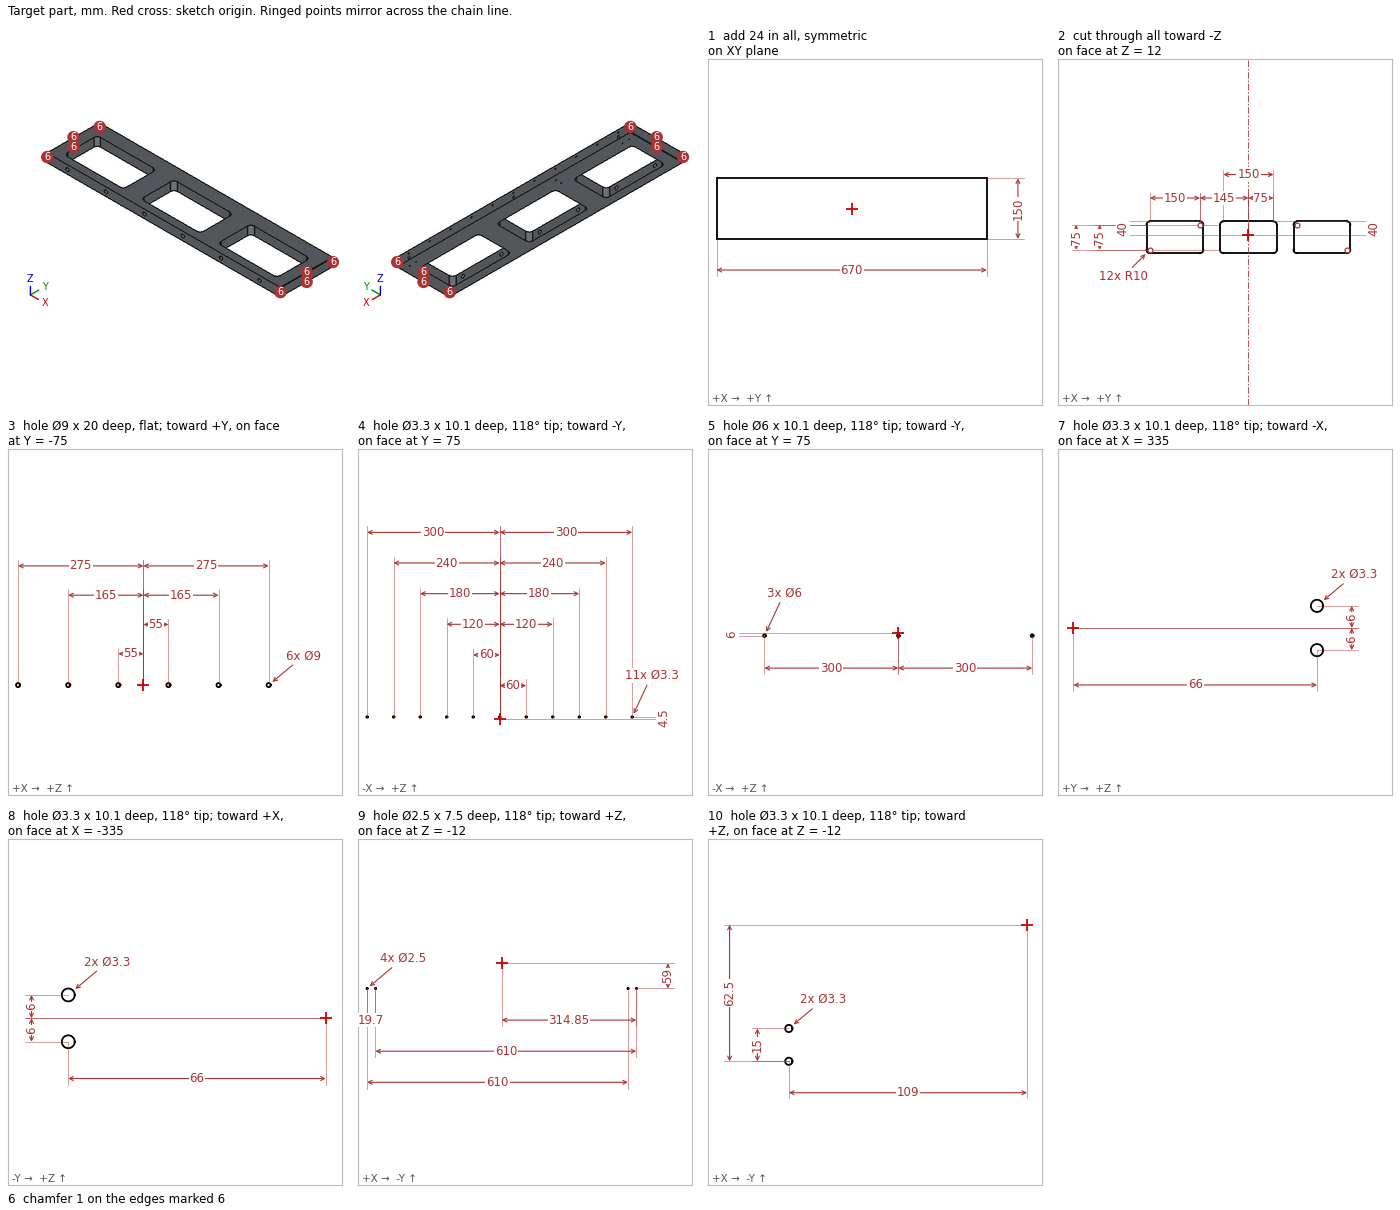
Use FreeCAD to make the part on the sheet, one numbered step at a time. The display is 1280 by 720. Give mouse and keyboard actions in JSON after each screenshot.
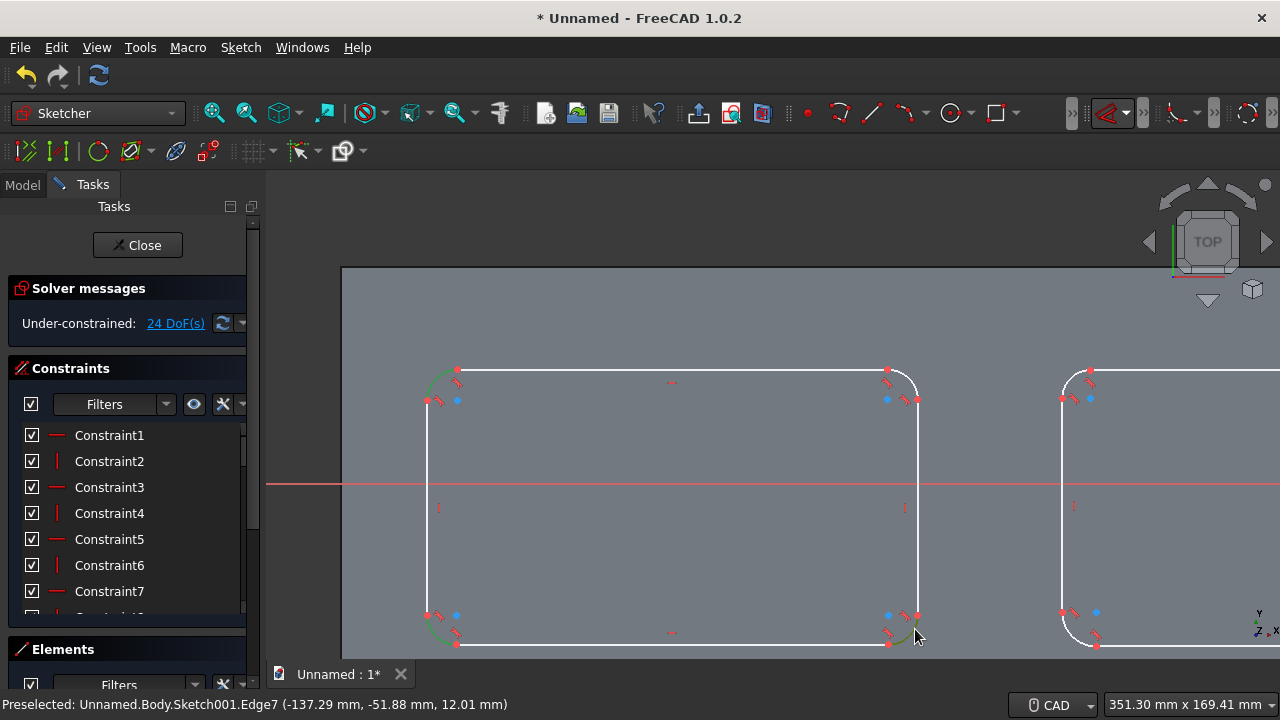
{"action": "left_click", "coordinate": [915, 386]}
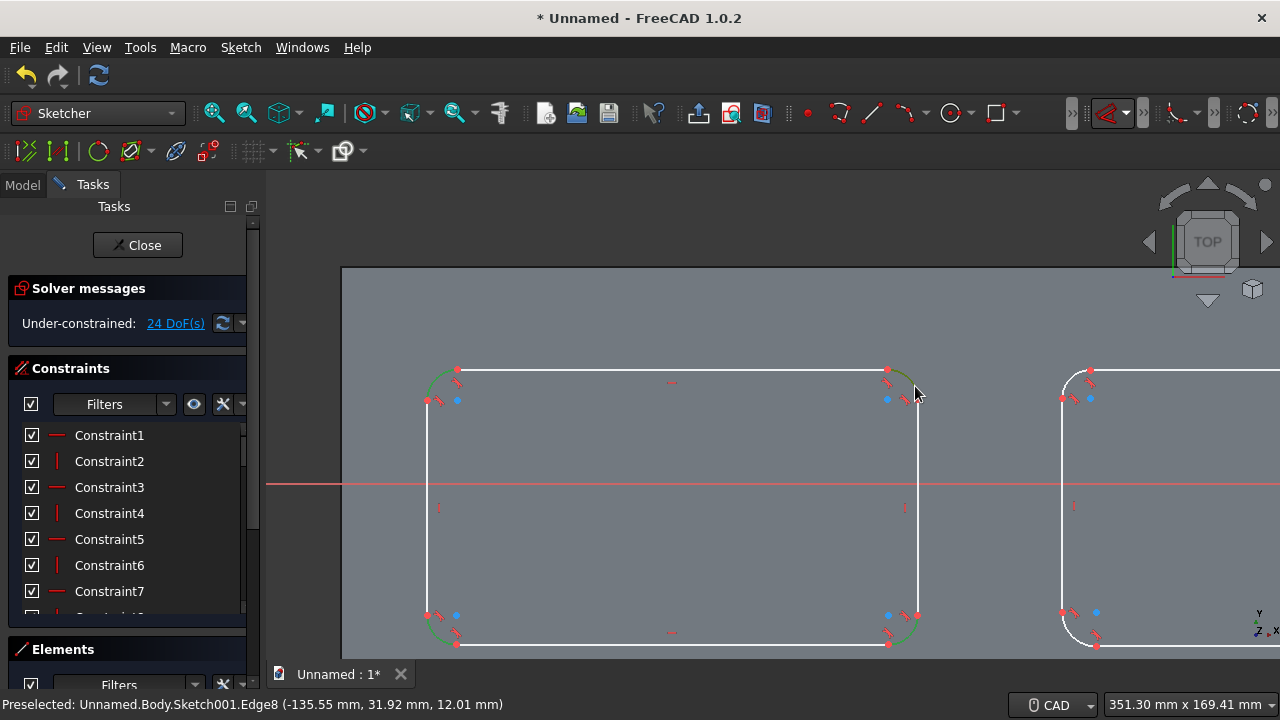
{"action": "left_click", "coordinate": [1078, 373]}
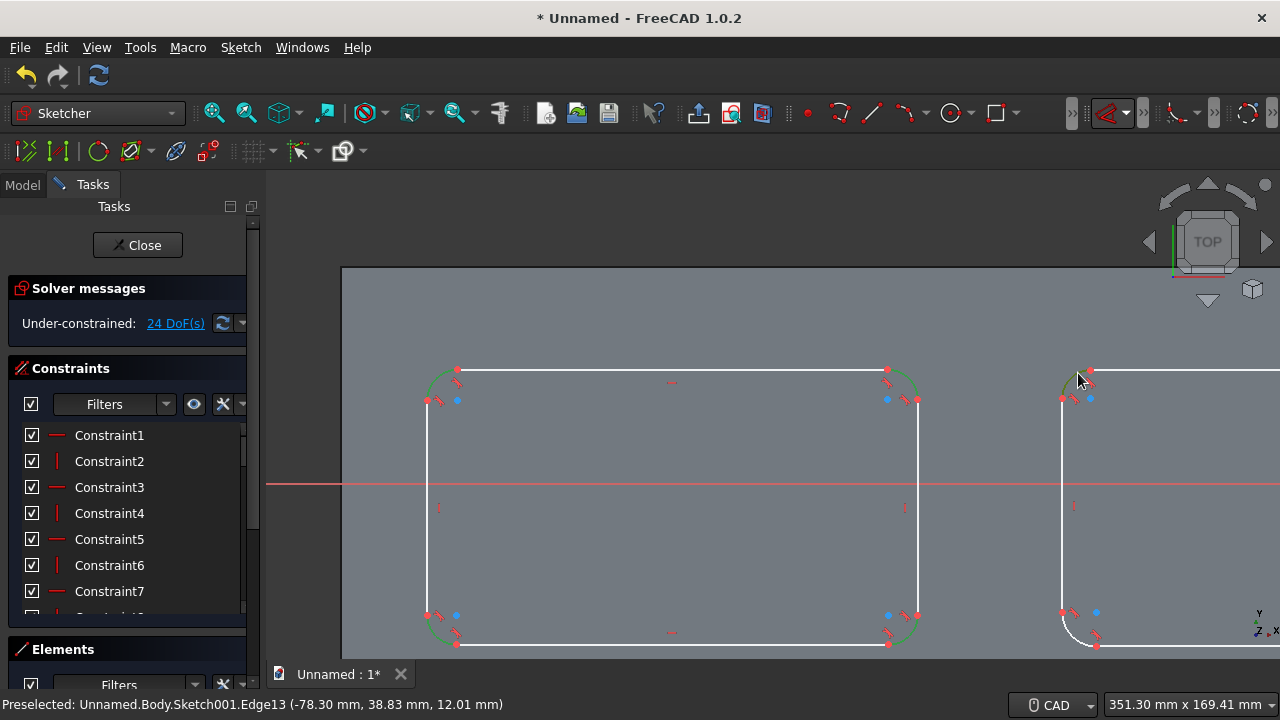
{"action": "left_click", "coordinate": [1066, 628]}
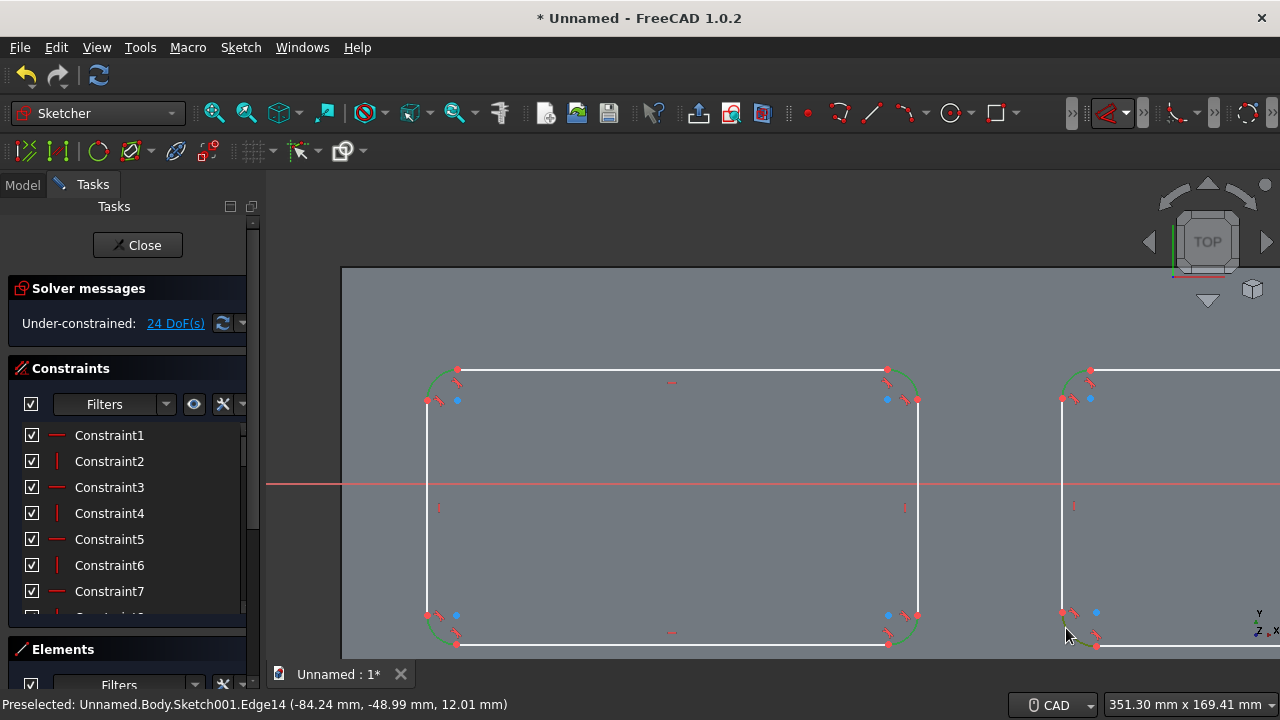
{"action": "scroll", "coordinate": [444, 375], "scroll_direction": "down", "scroll_amount": 6}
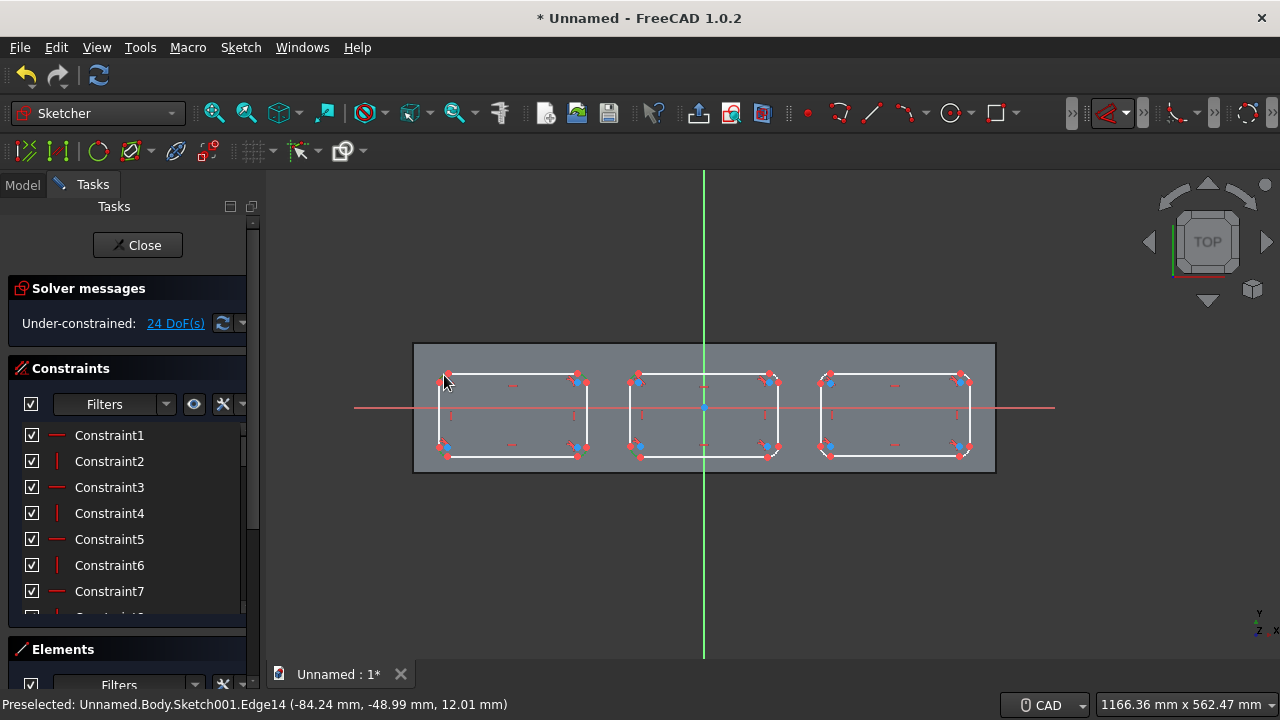
{"action": "scroll", "coordinate": [773, 456], "scroll_direction": "up", "scroll_amount": 6}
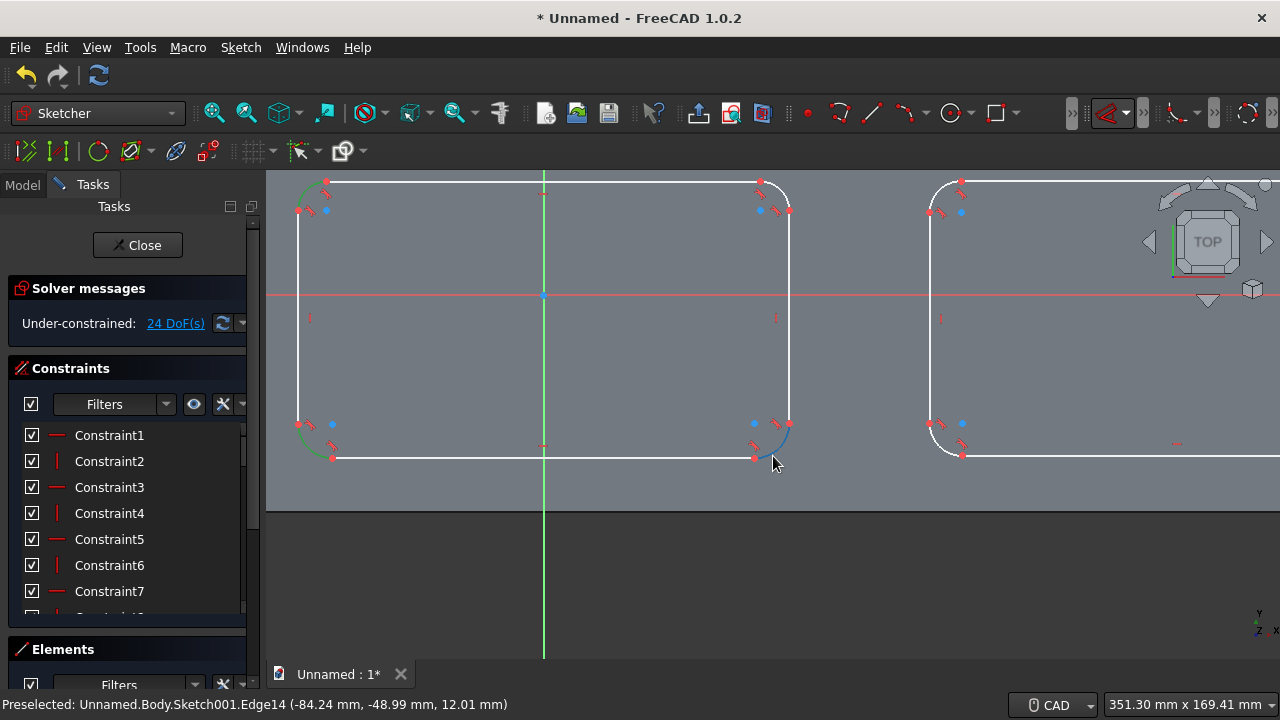
{"action": "left_click", "coordinate": [770, 454]}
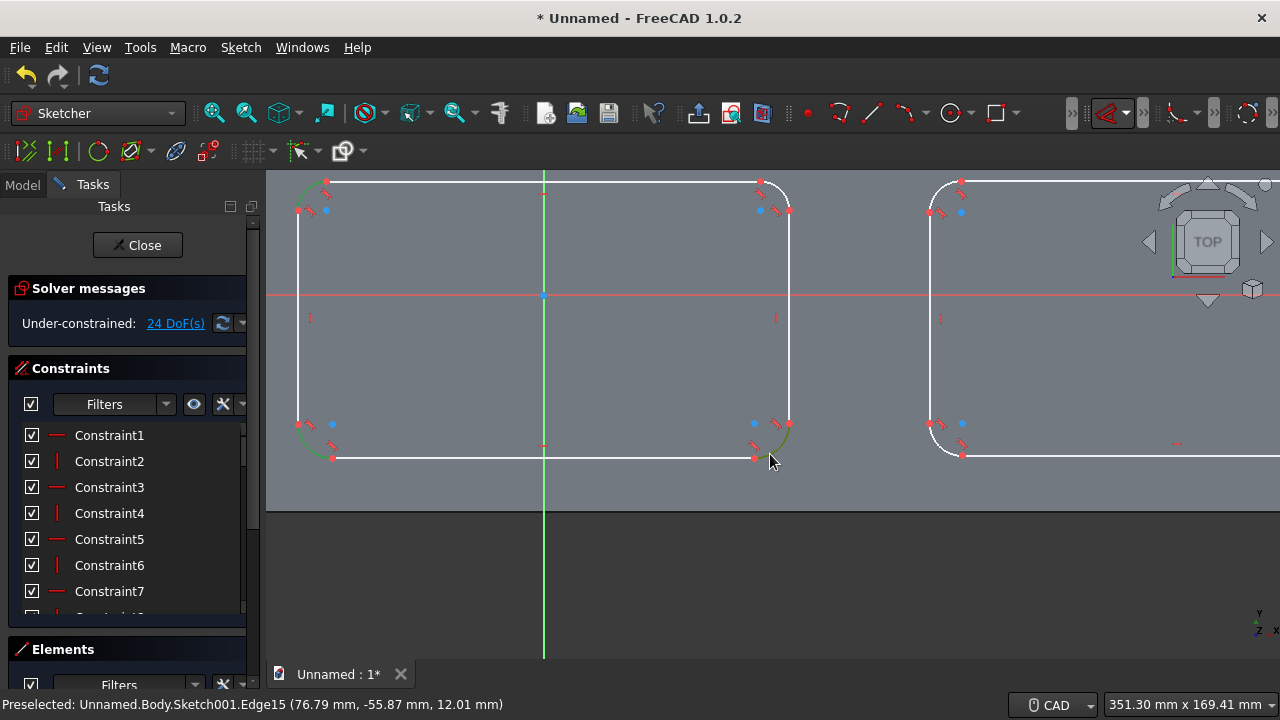
{"action": "scroll", "coordinate": [774, 457], "scroll_direction": "down", "scroll_amount": 6}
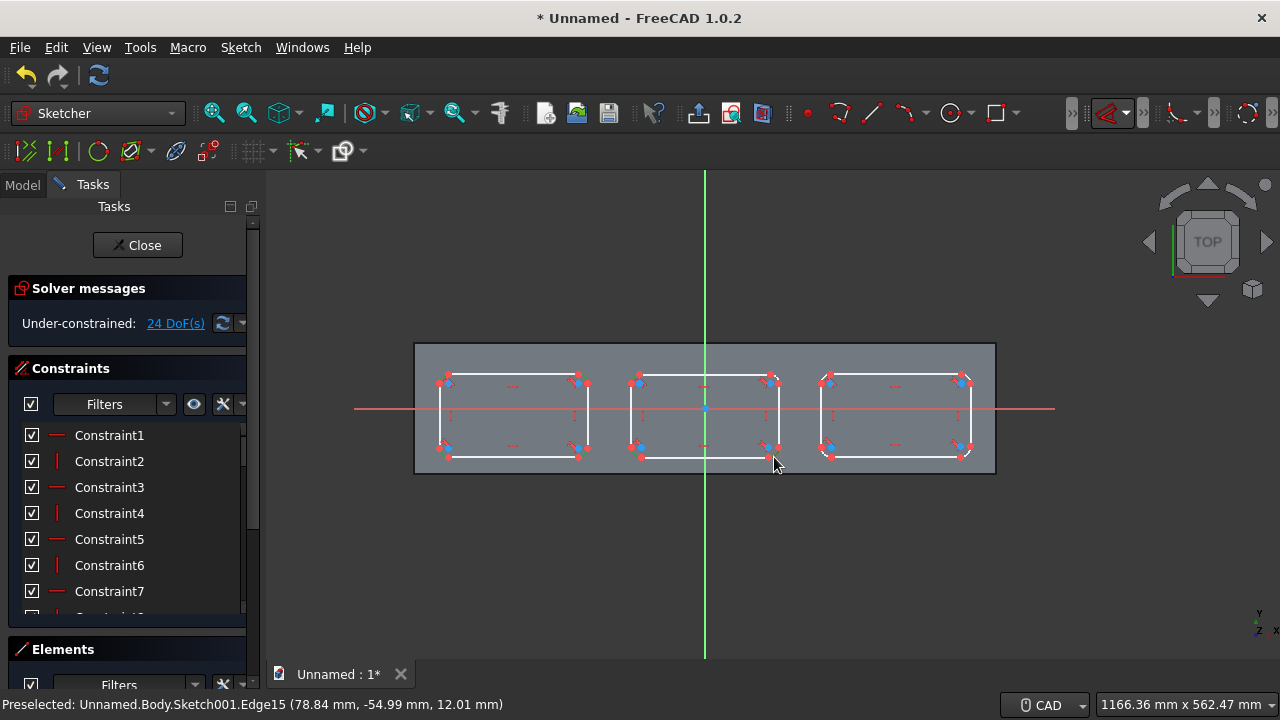
{"action": "scroll", "coordinate": [778, 379], "scroll_direction": "up", "scroll_amount": 7}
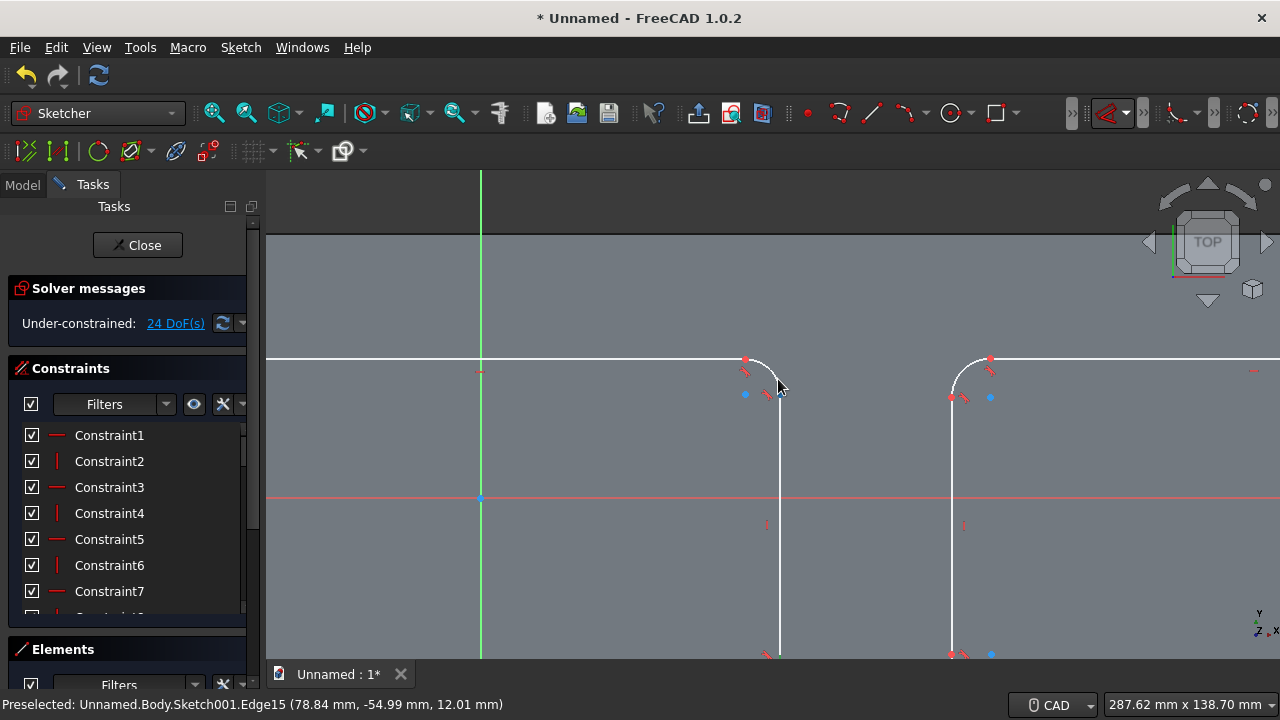
{"action": "left_click", "coordinate": [776, 378]}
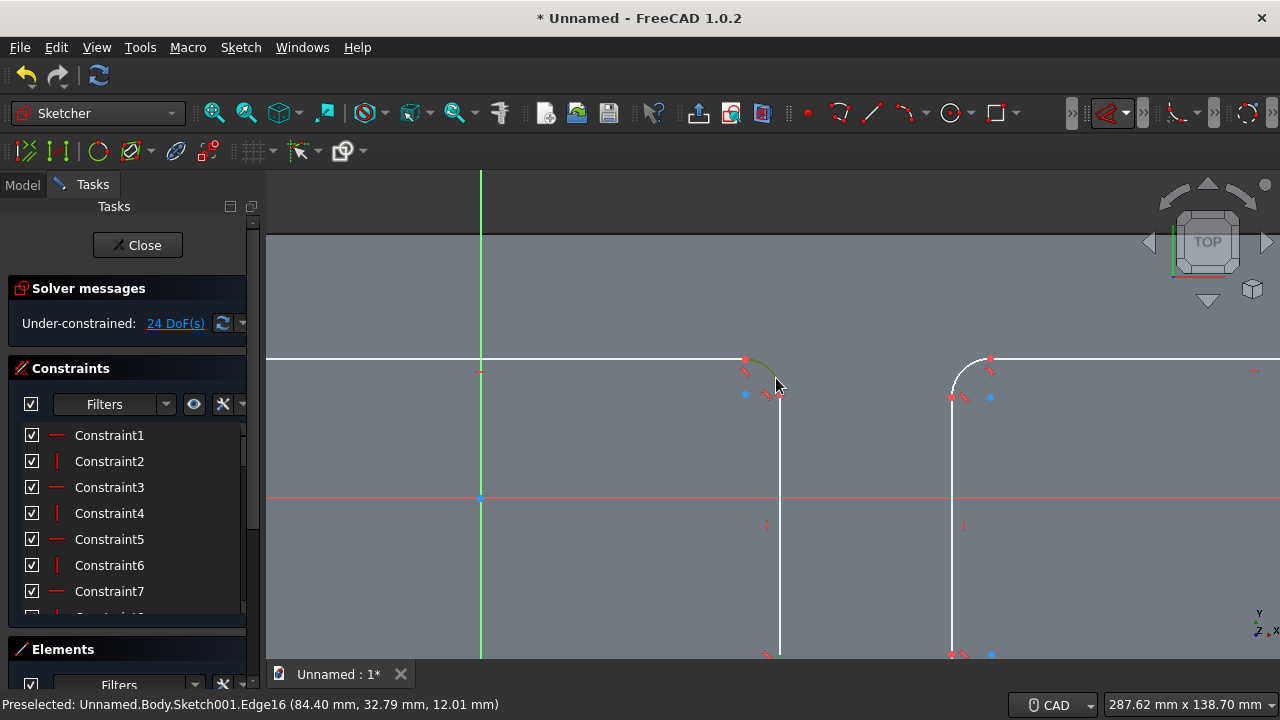
{"action": "left_click", "coordinate": [973, 363]}